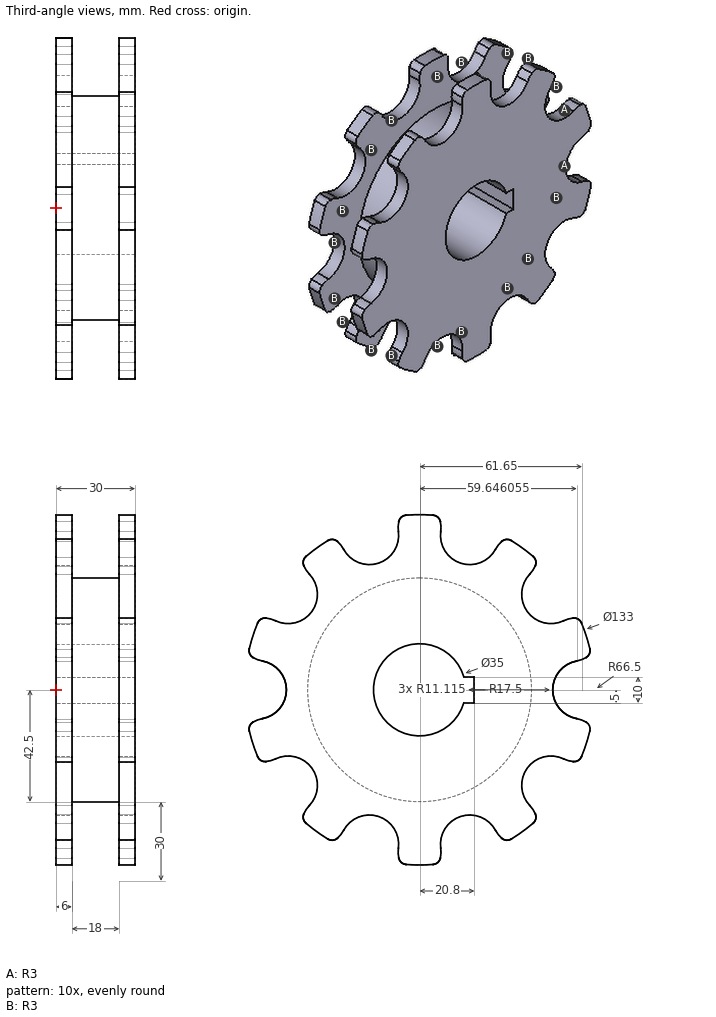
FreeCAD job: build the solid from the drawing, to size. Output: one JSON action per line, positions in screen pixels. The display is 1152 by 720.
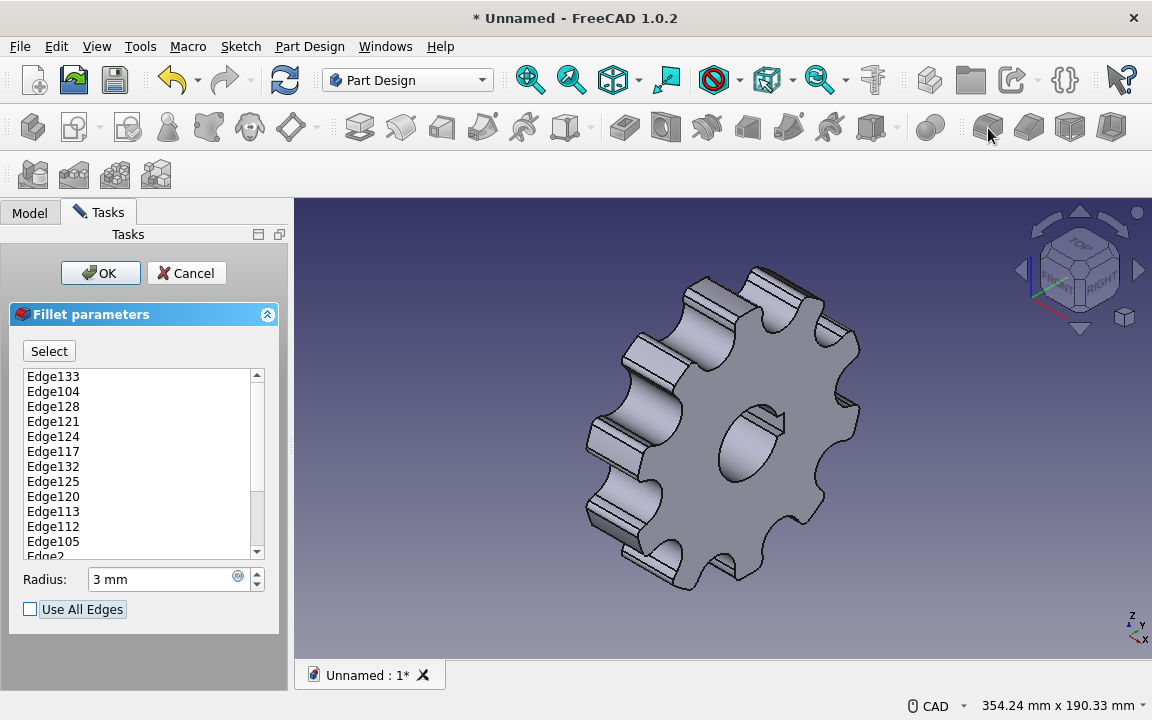
{"action": "left_click", "coordinate": [101, 273]}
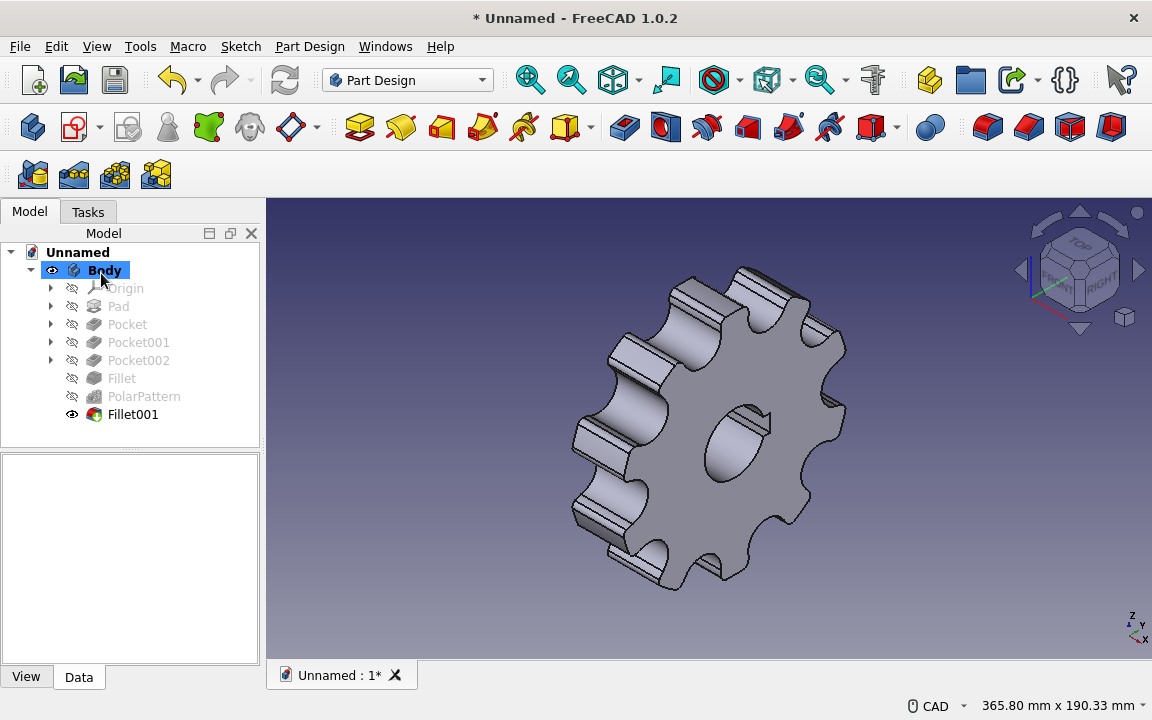
{"action": "left_click", "coordinate": [74, 128]}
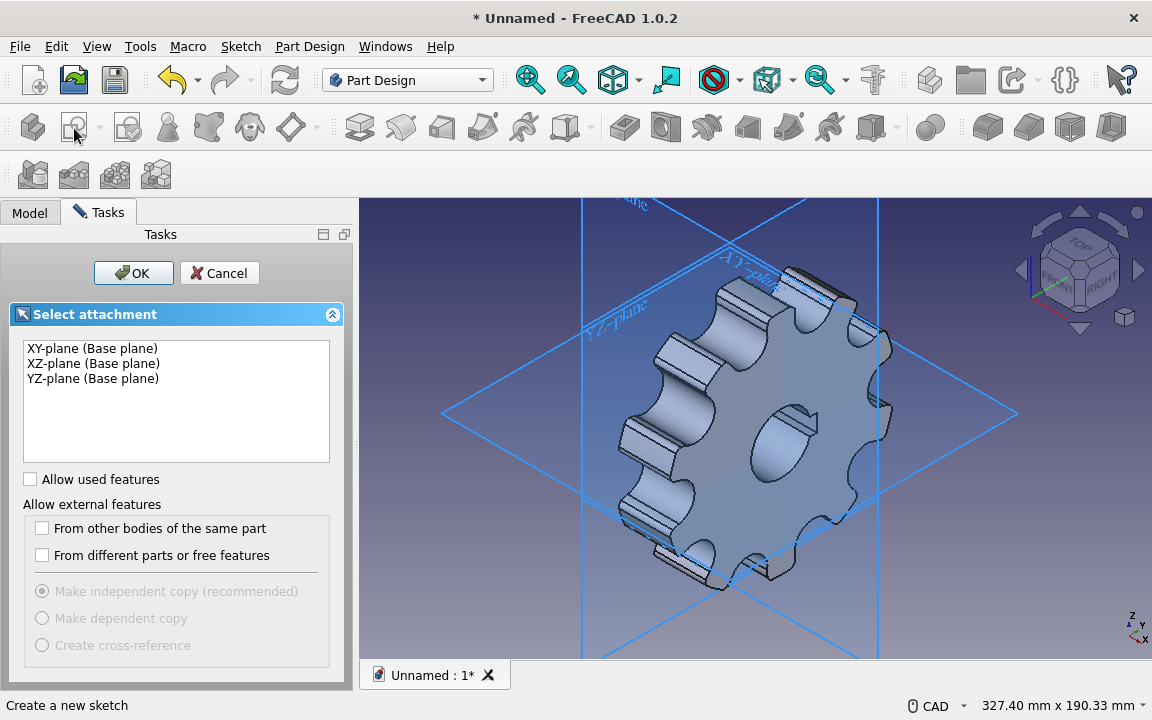
{"action": "left_click", "coordinate": [84, 364]}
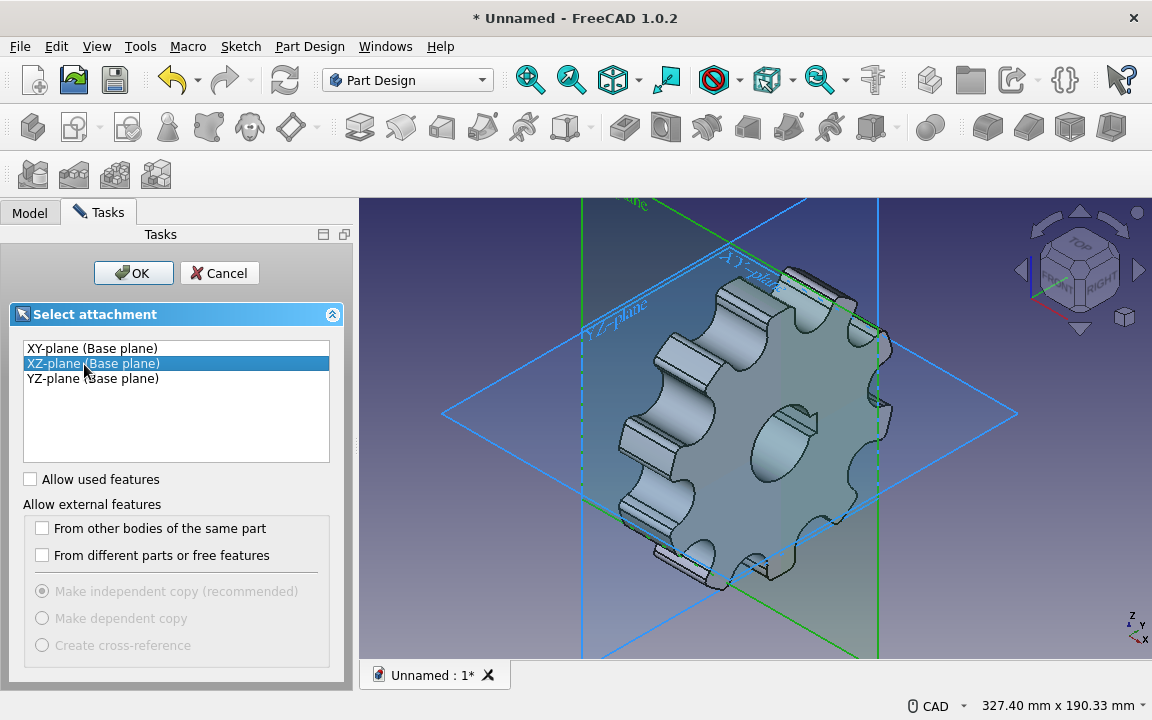
{"action": "left_click", "coordinate": [134, 273]}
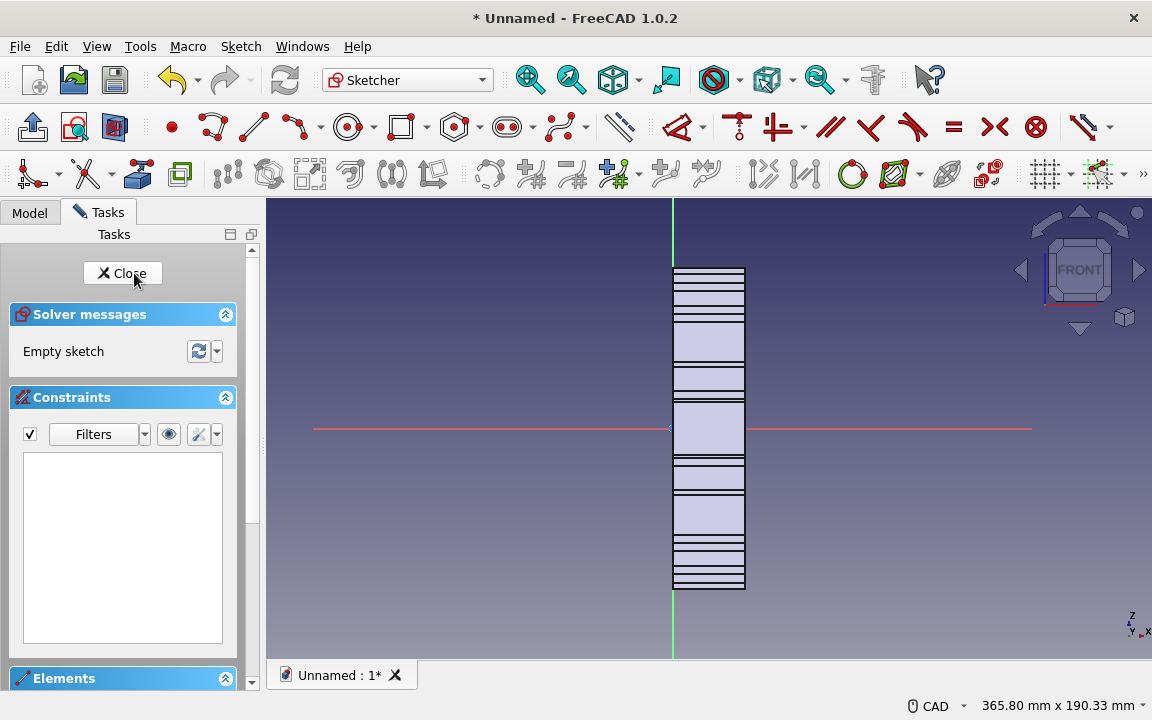
{"action": "left_click", "coordinate": [115, 128]}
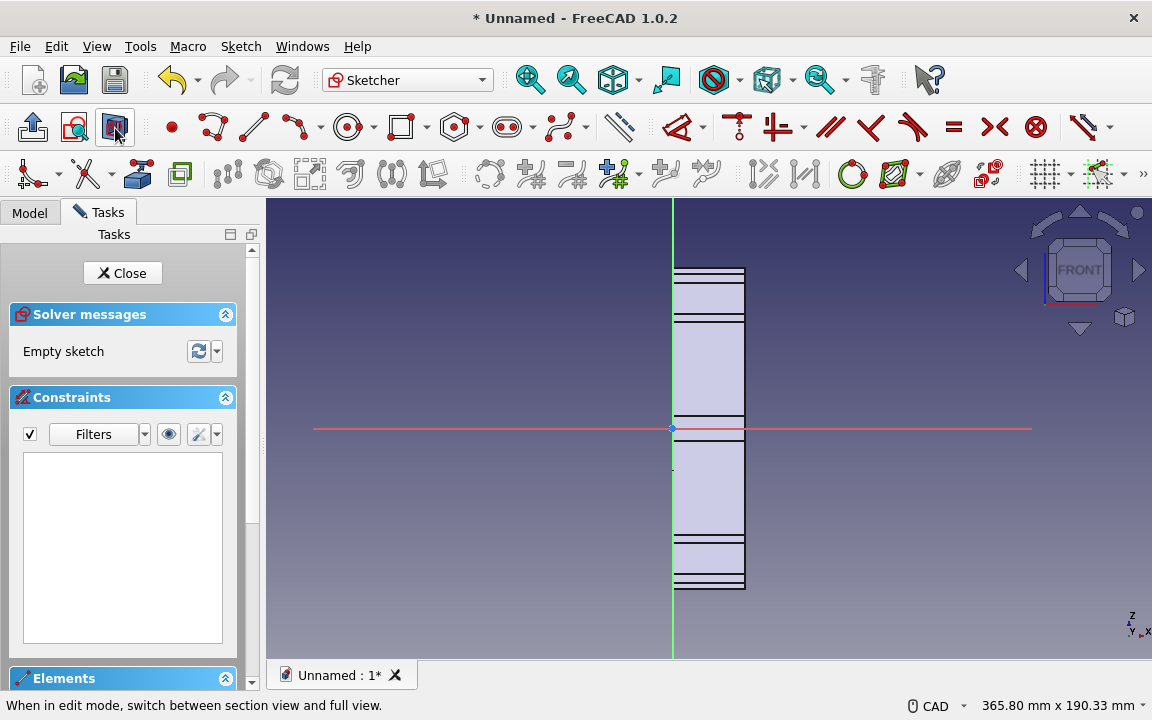
{"action": "scroll", "coordinate": [826, 631], "scroll_direction": "up", "scroll_amount": 2}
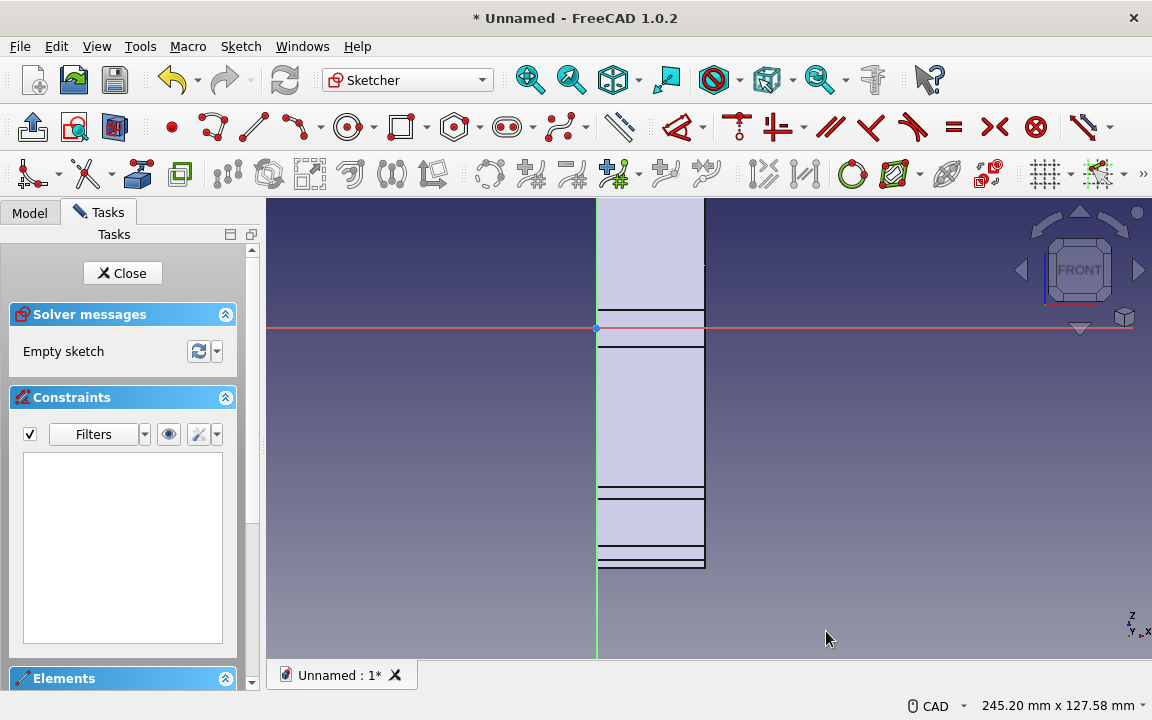
{"action": "left_click", "coordinate": [400, 128]}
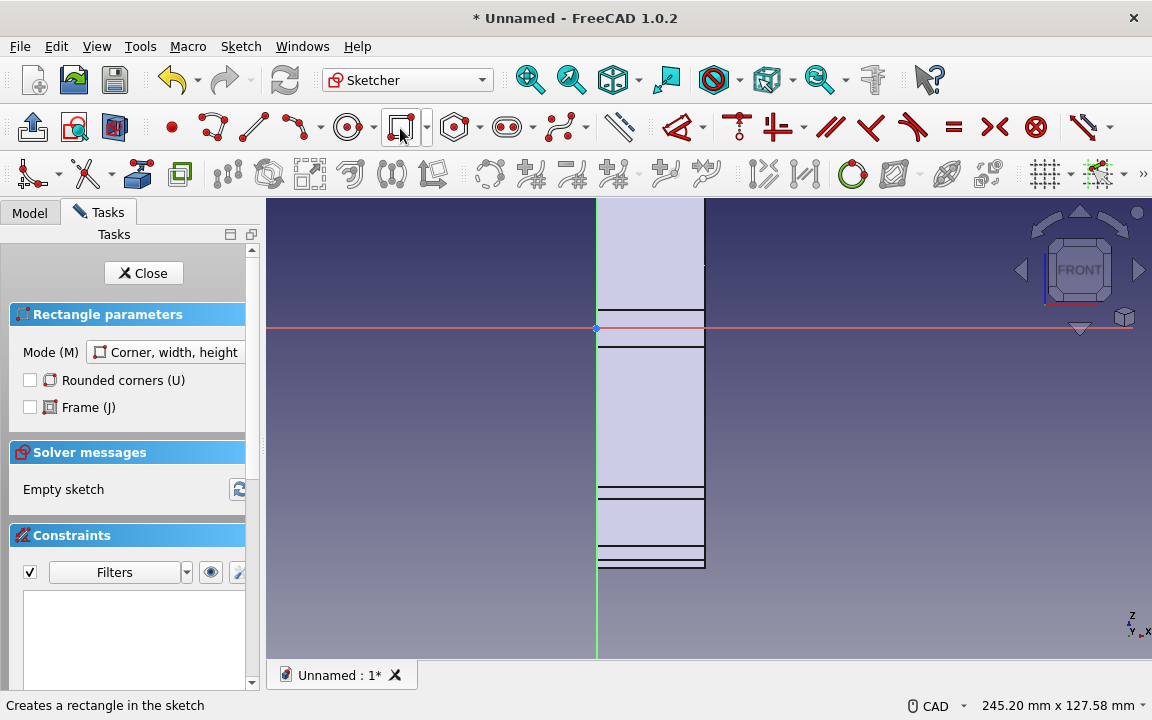
{"action": "left_click", "coordinate": [619, 482]}
{"action": "mouse_move", "coordinate": [684, 590]}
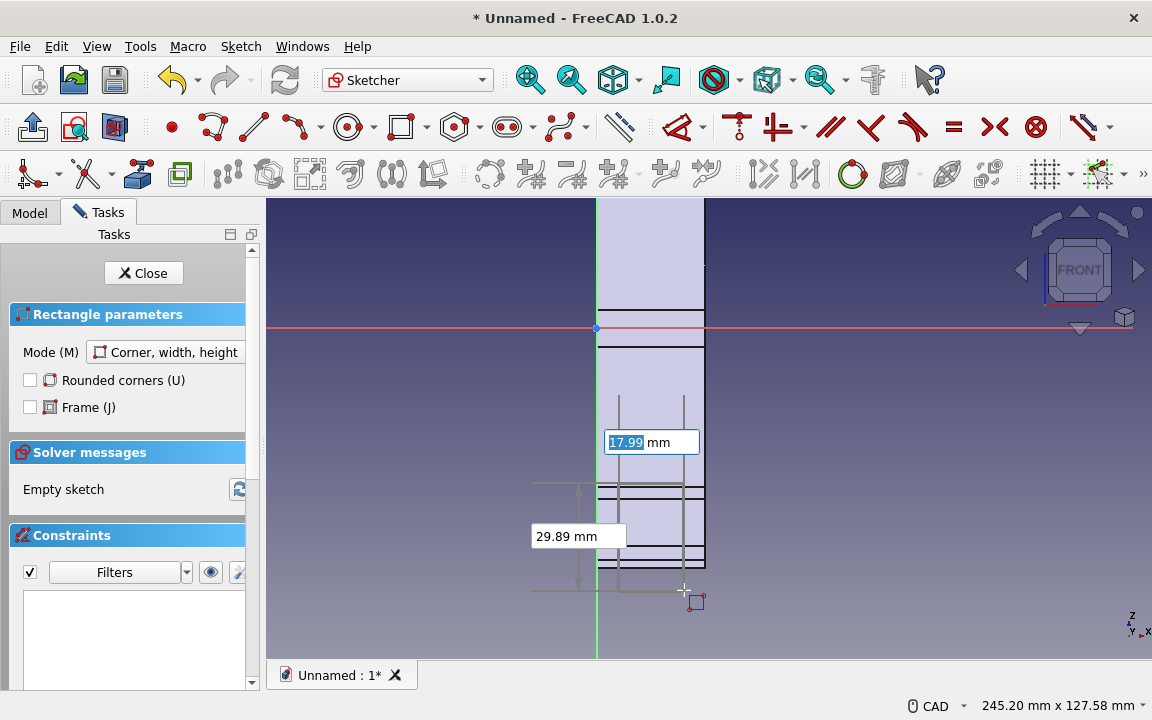
{"action": "type", "text": "18"}
{"action": "key", "text": "Tab"}
{"action": "type", "text": "30"}
{"action": "key", "text": "Return"}
{"action": "key", "text": "Escape"}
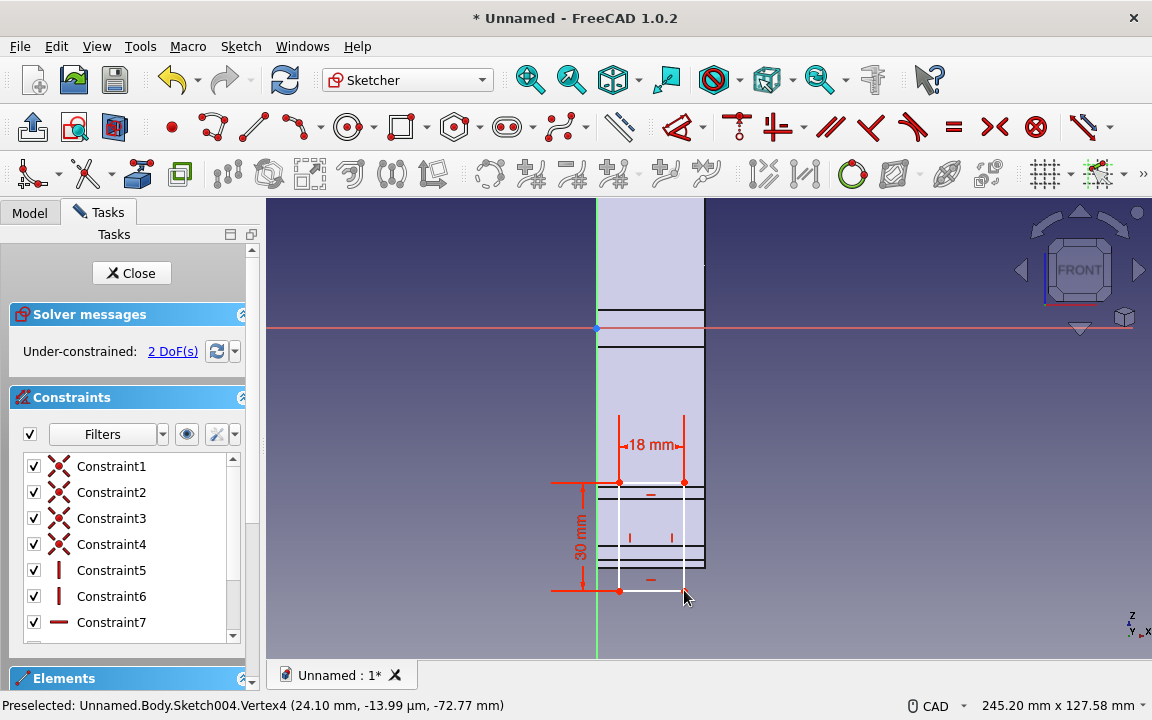
{"action": "left_click", "coordinate": [676, 128]}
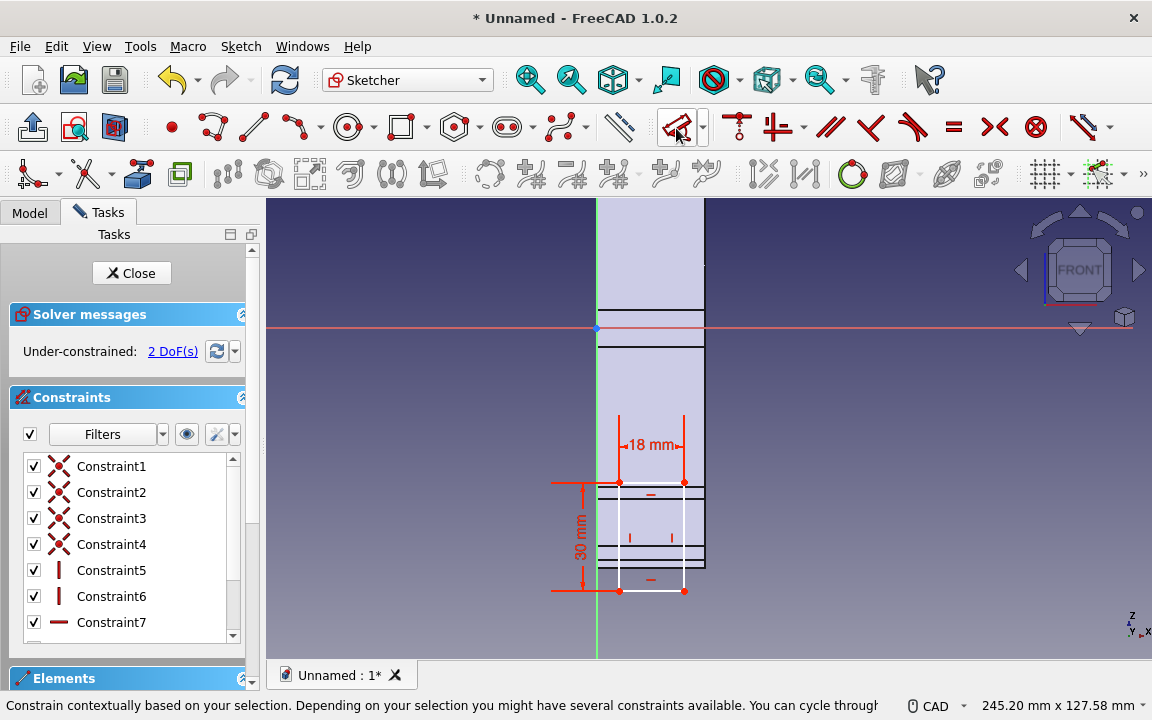
{"action": "scroll", "coordinate": [619, 483], "scroll_direction": "up", "scroll_amount": 4}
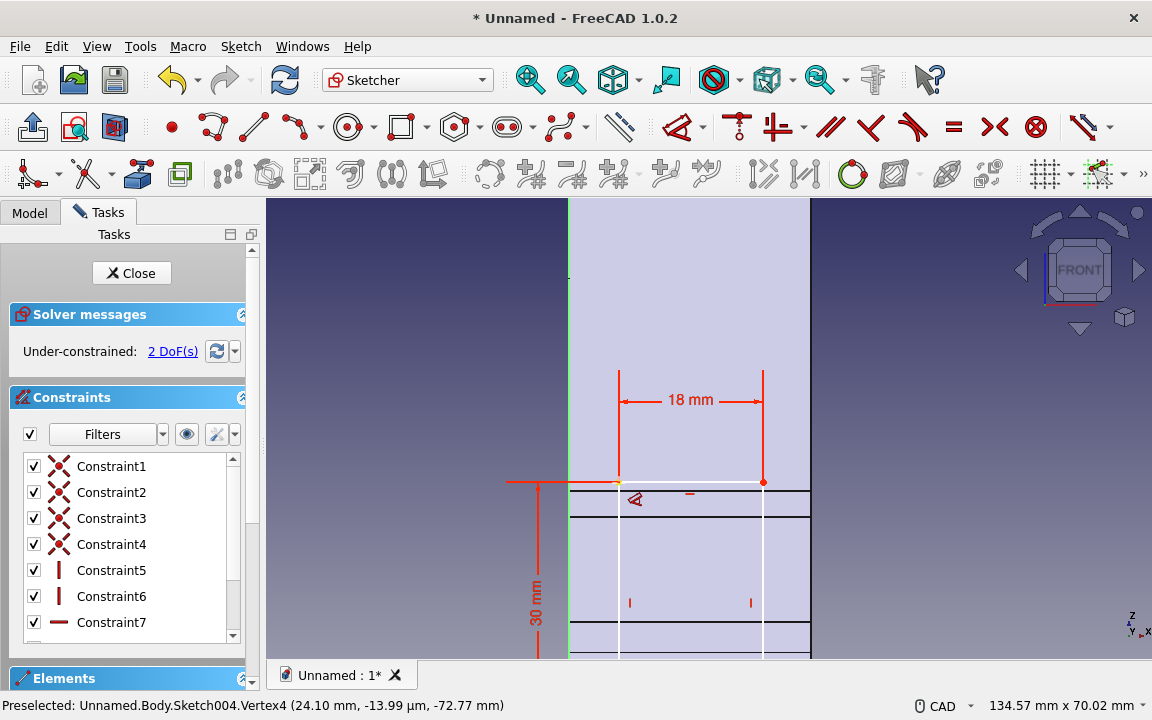
{"action": "left_click", "coordinate": [619, 482]}
{"action": "left_click", "coordinate": [594, 516]}